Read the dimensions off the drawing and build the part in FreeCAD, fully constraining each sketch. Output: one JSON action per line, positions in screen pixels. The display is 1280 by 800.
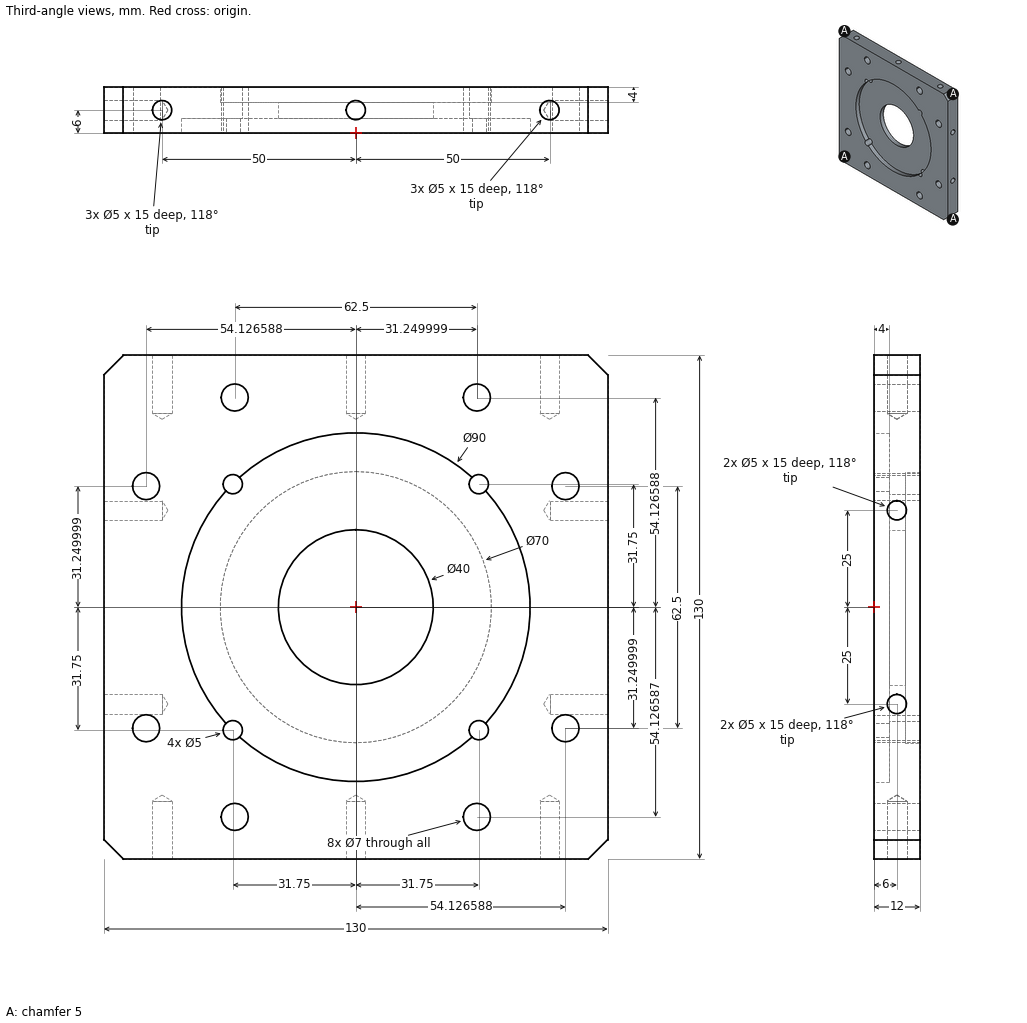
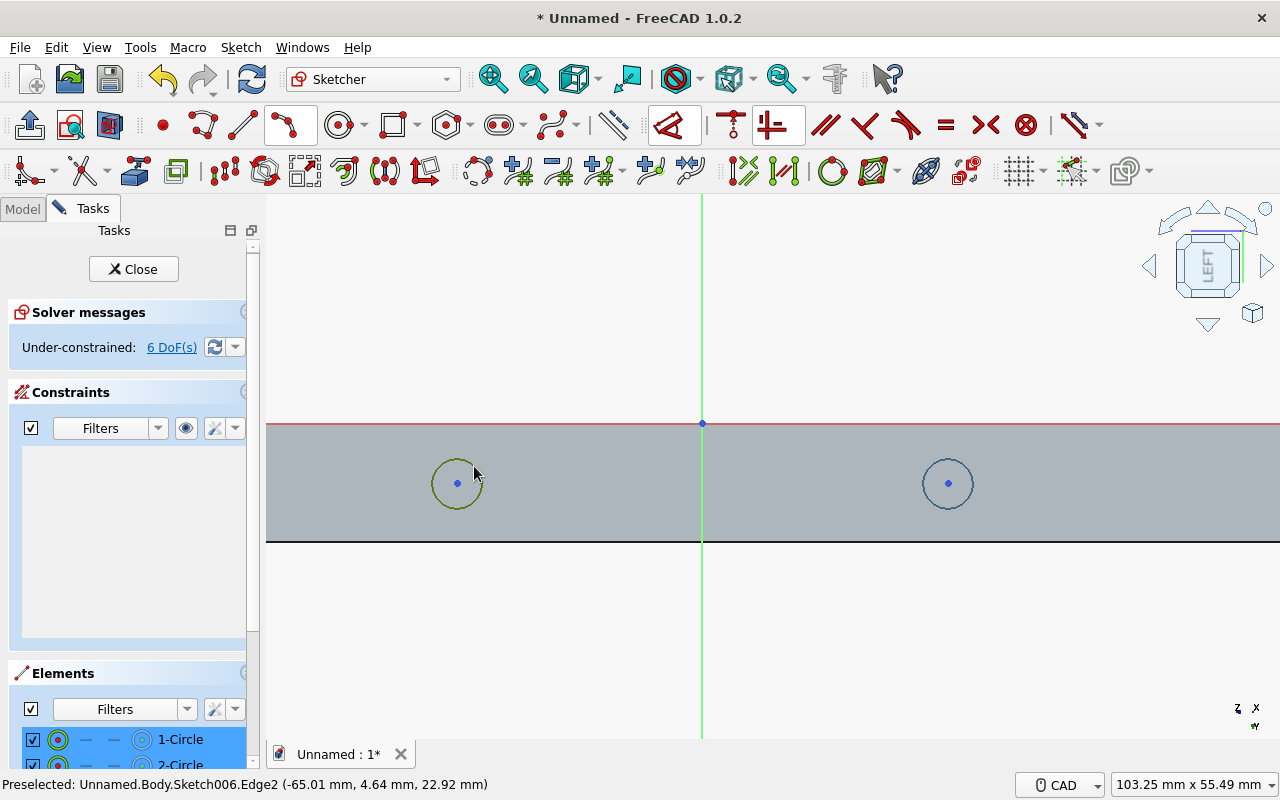
{"action": "key", "text": "e"}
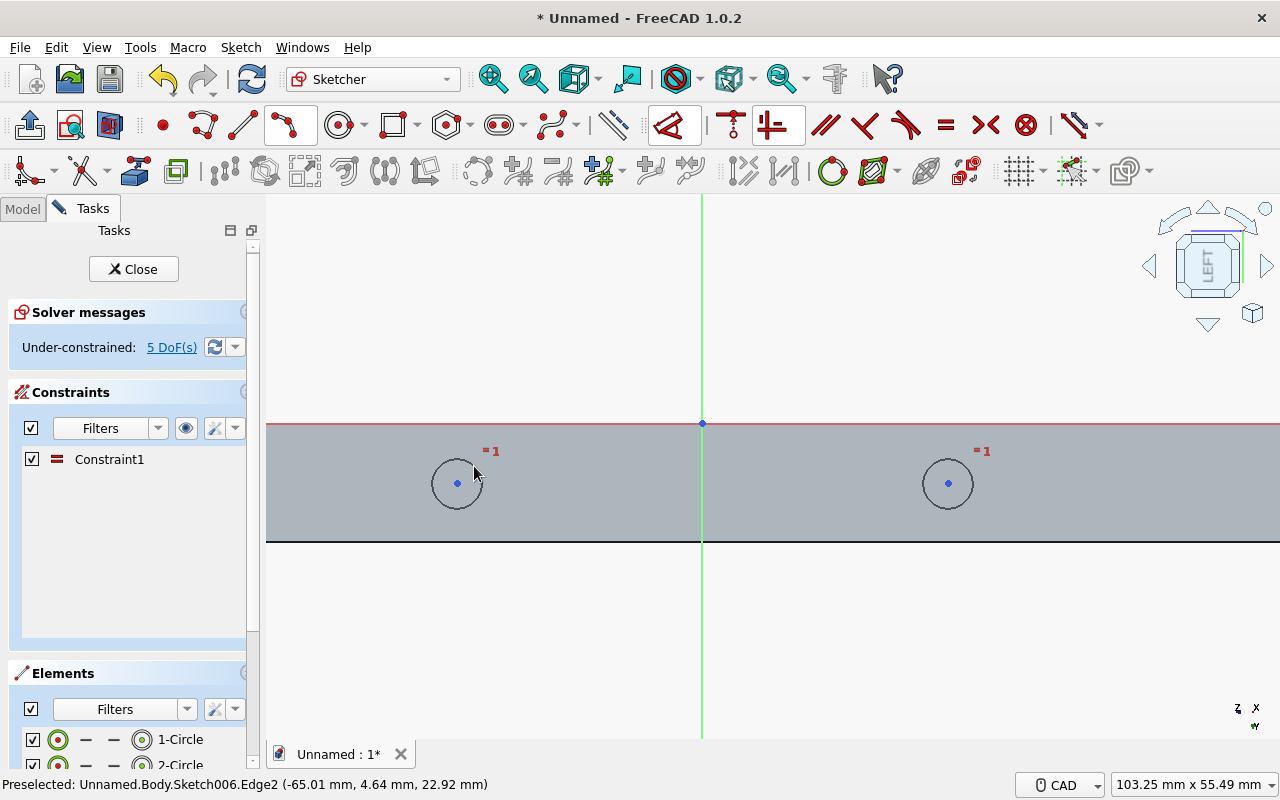
{"action": "left_click", "coordinate": [948, 484]}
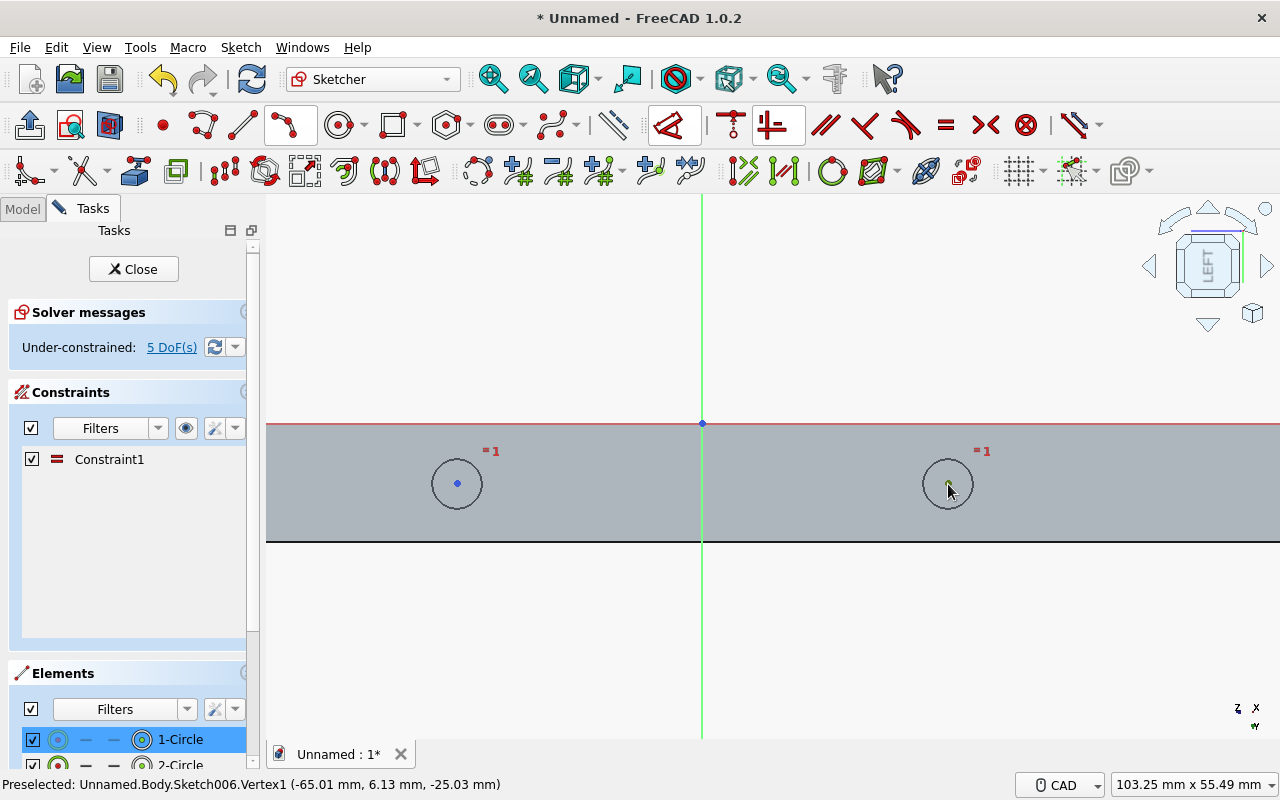
{"action": "left_click", "coordinate": [457, 484]}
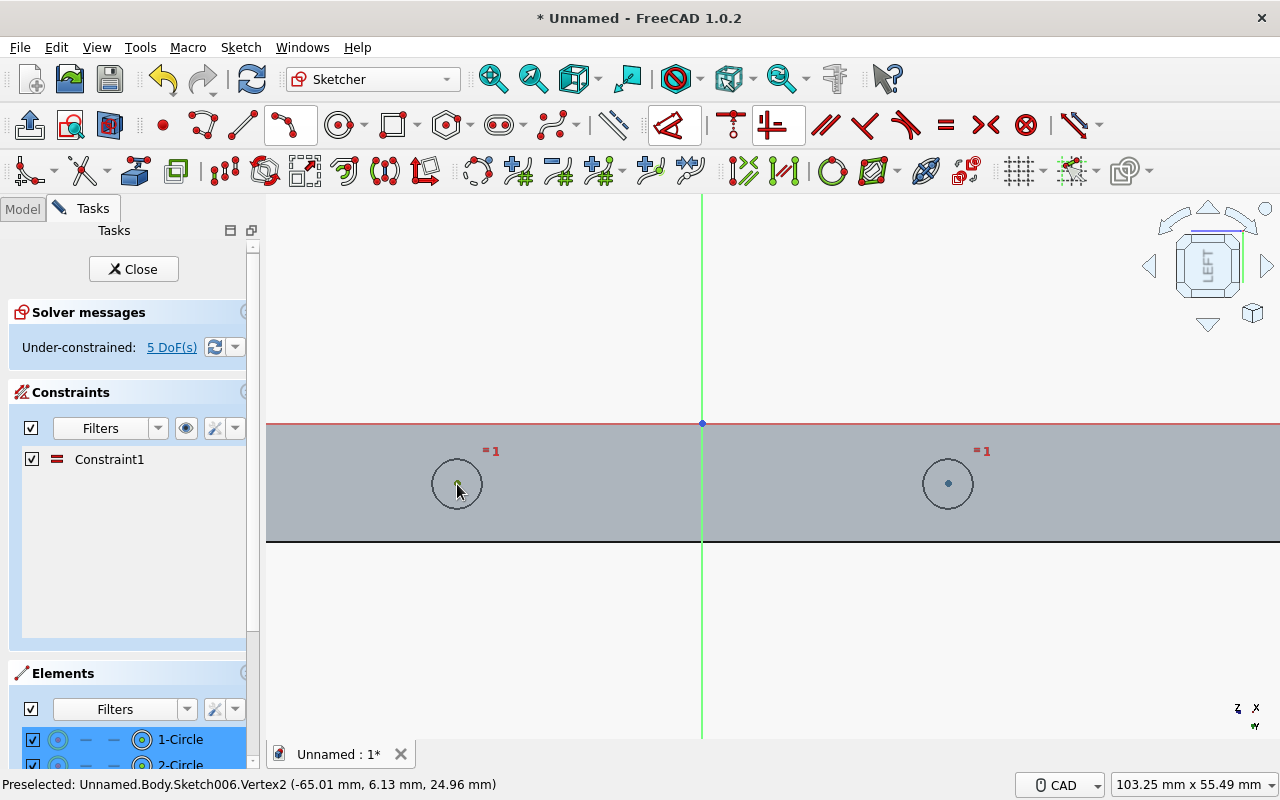
{"action": "key", "text": "h"}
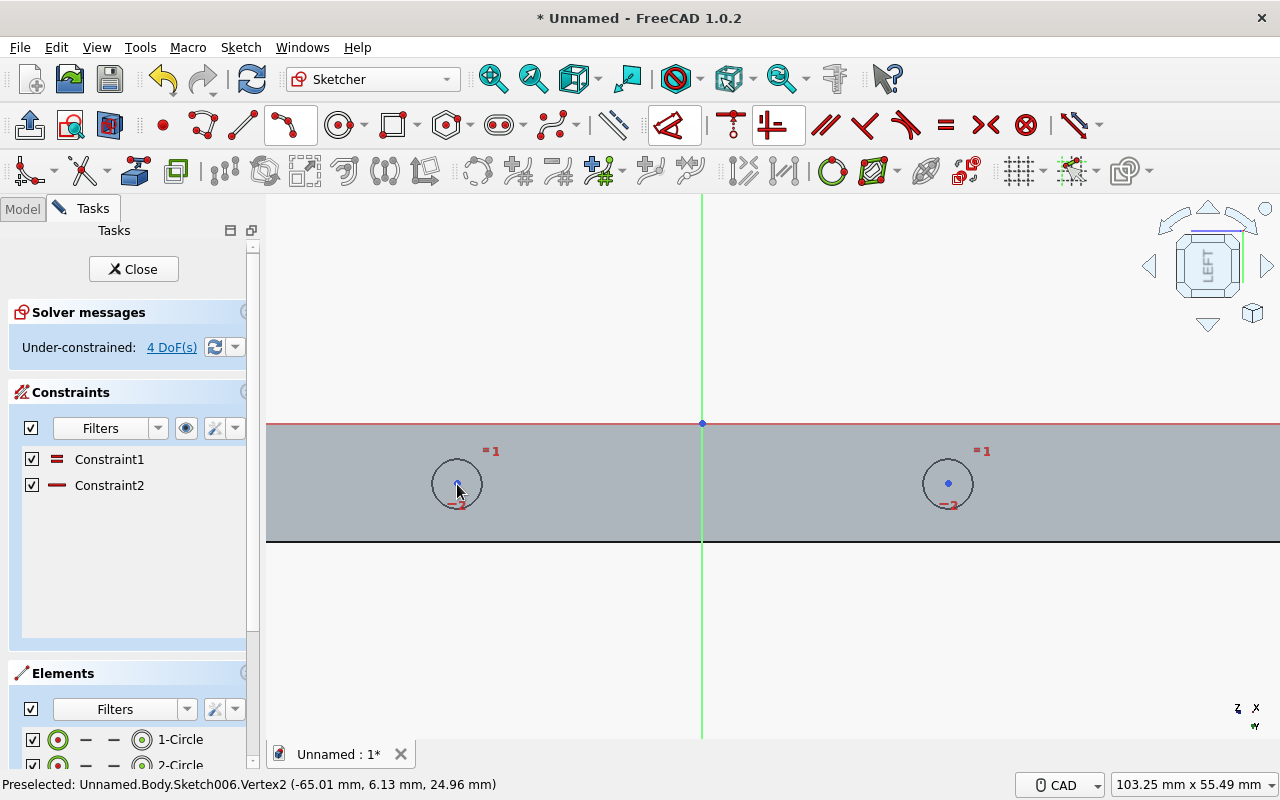
{"action": "key", "text": "d"}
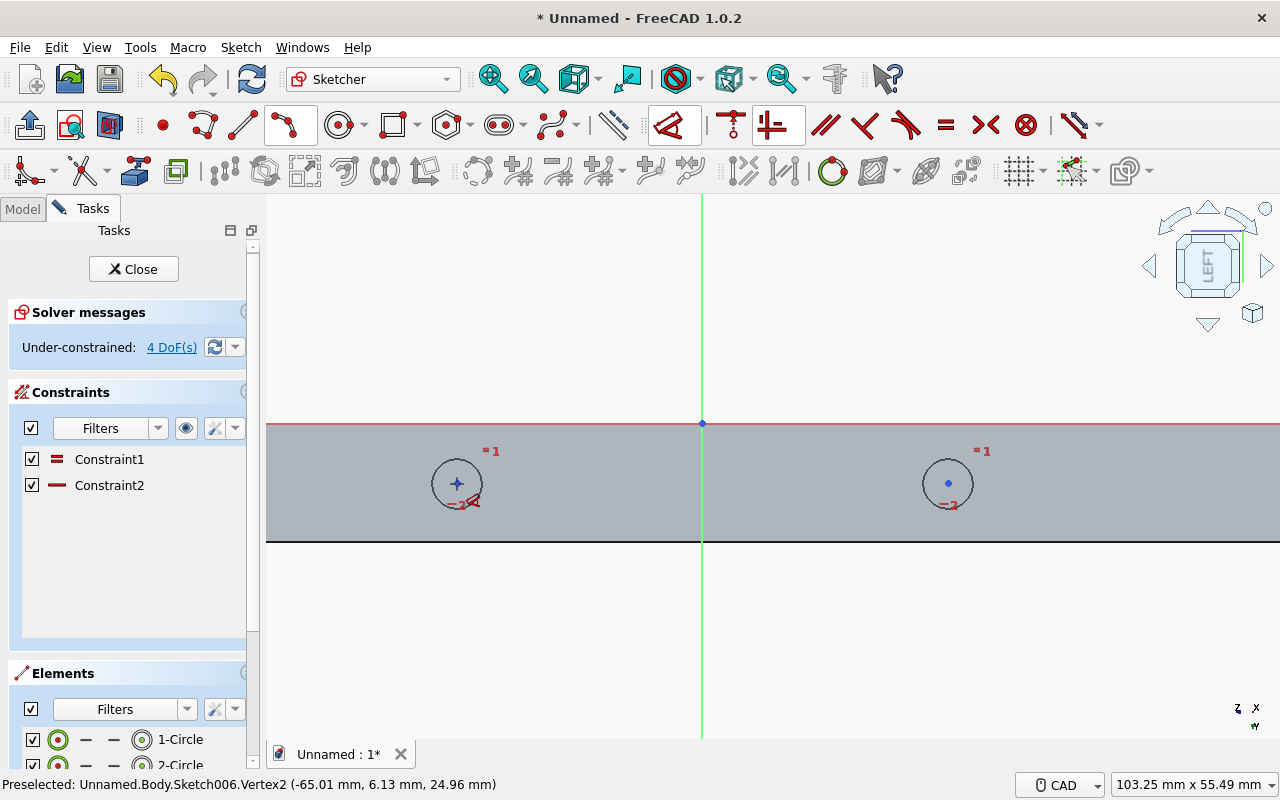
{"action": "left_click", "coordinate": [965, 466]}
{"action": "left_click", "coordinate": [987, 443]}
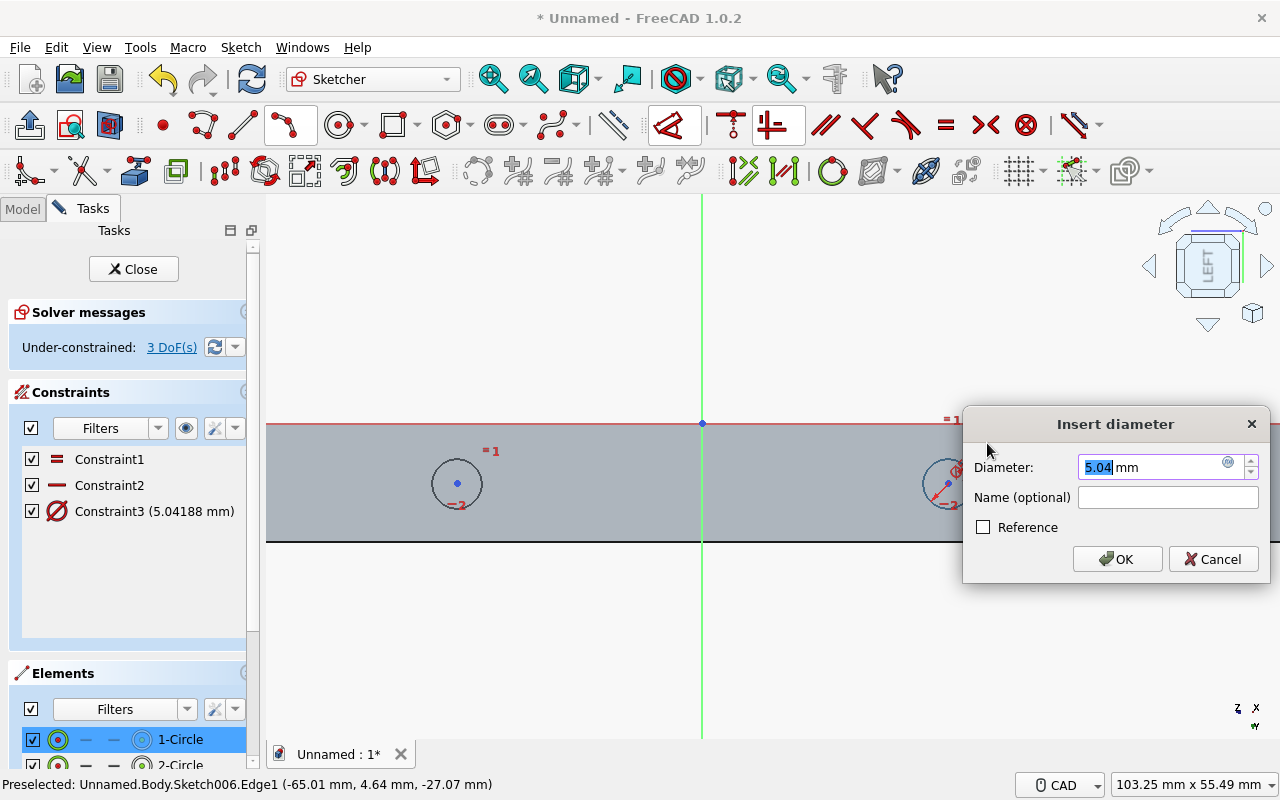
{"action": "type", "text": "5"}
{"action": "key", "text": "Return"}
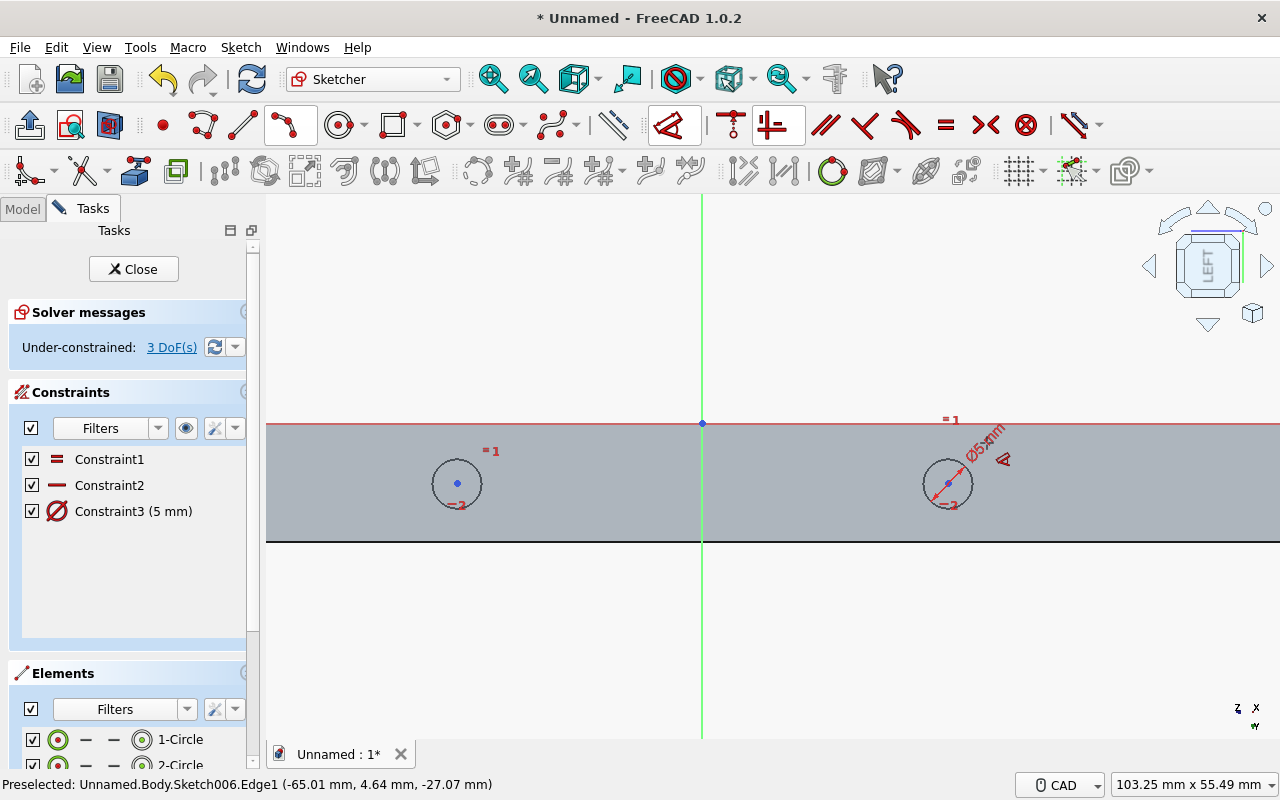
{"action": "left_click", "coordinate": [948, 484]}
{"action": "left_click", "coordinate": [982, 468]}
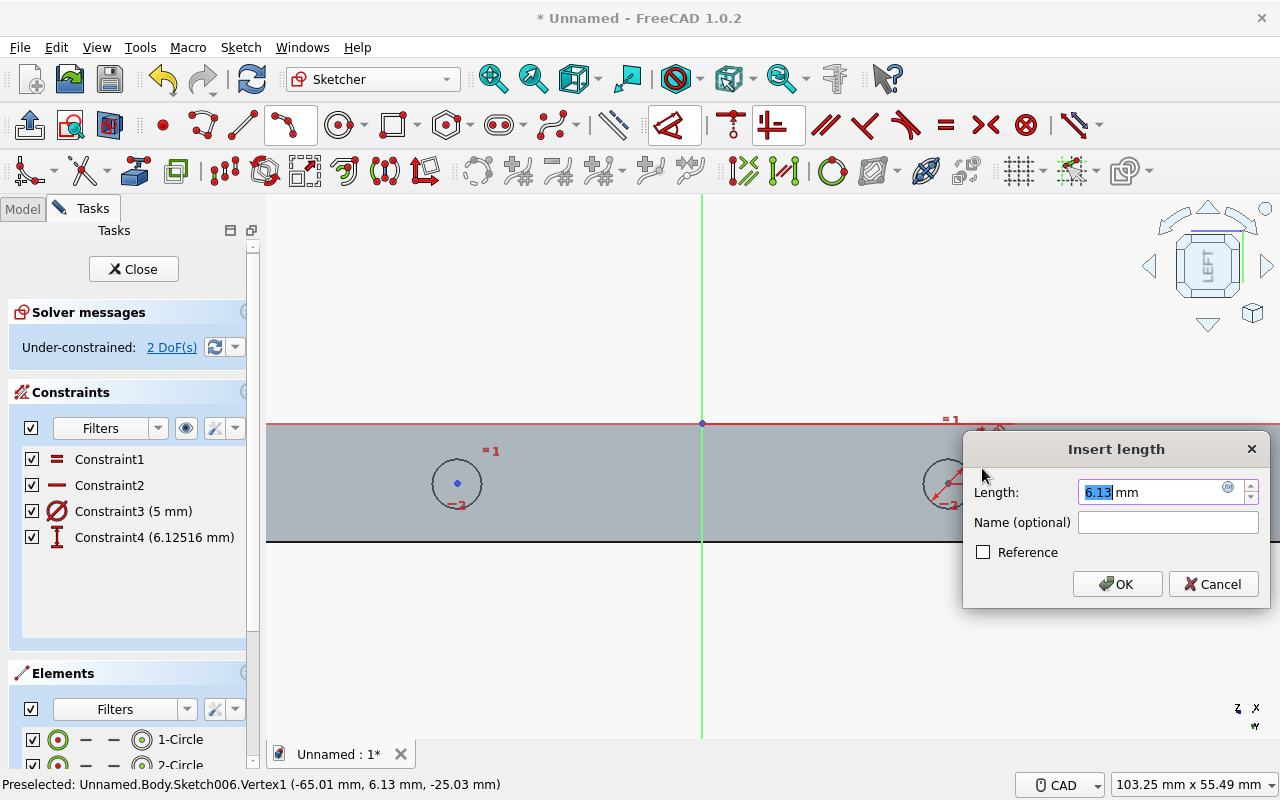
{"action": "type", "text": "6"}
{"action": "key", "text": "Return"}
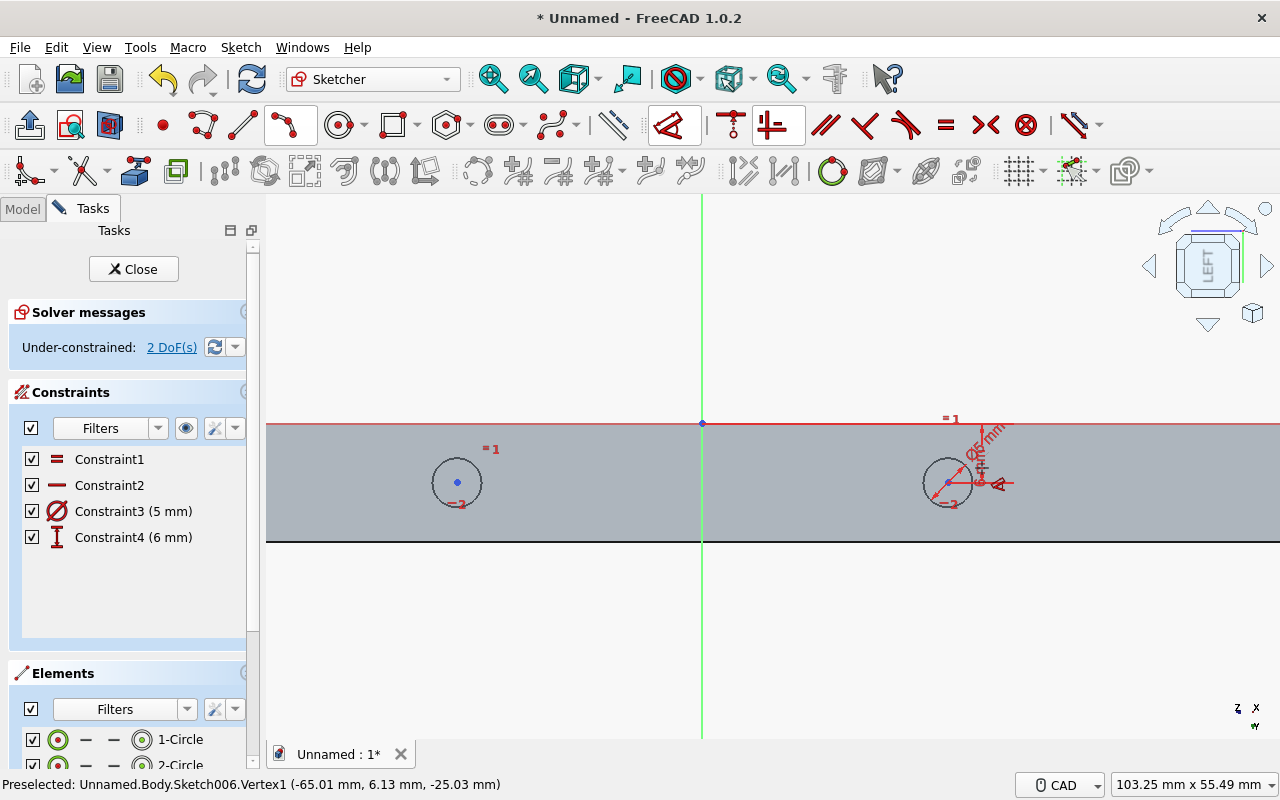
{"action": "left_click", "coordinate": [948, 483]}
{"action": "left_click", "coordinate": [825, 390]}